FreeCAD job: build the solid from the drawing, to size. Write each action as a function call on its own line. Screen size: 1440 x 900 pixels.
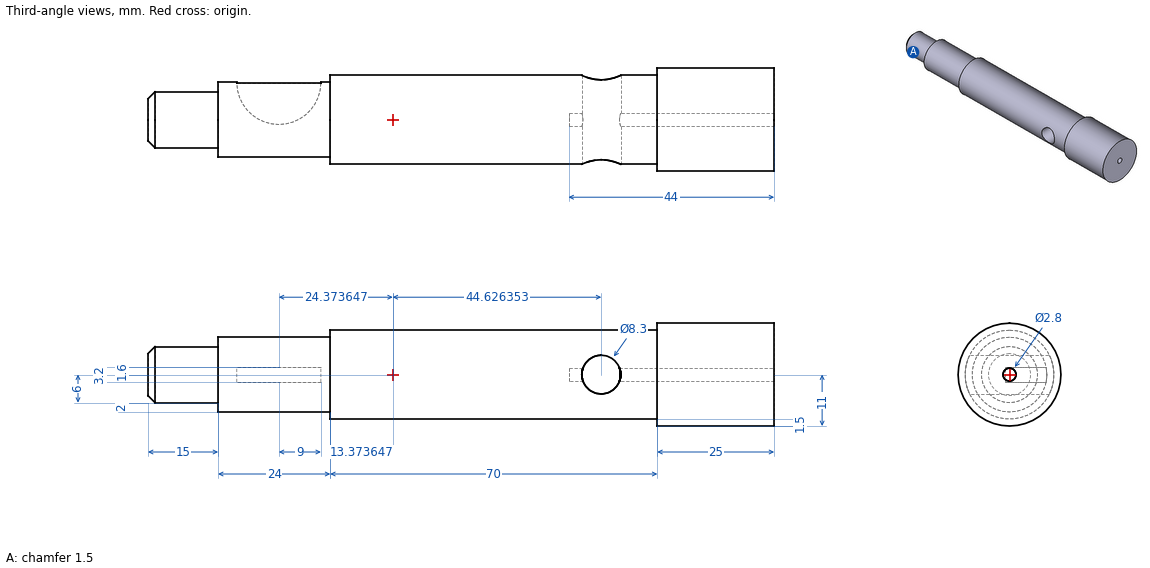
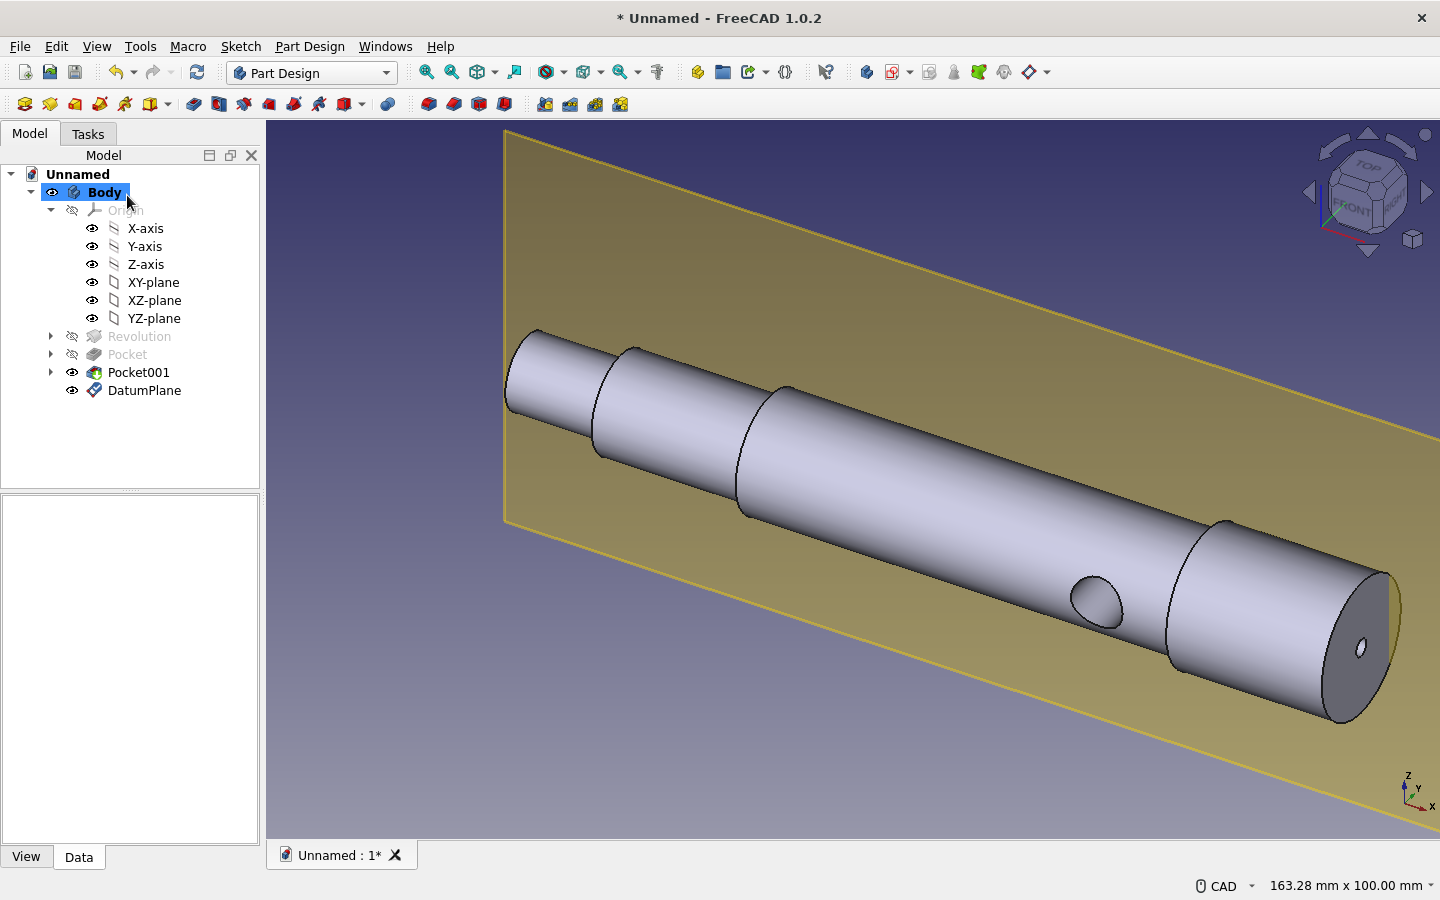
click(117, 390)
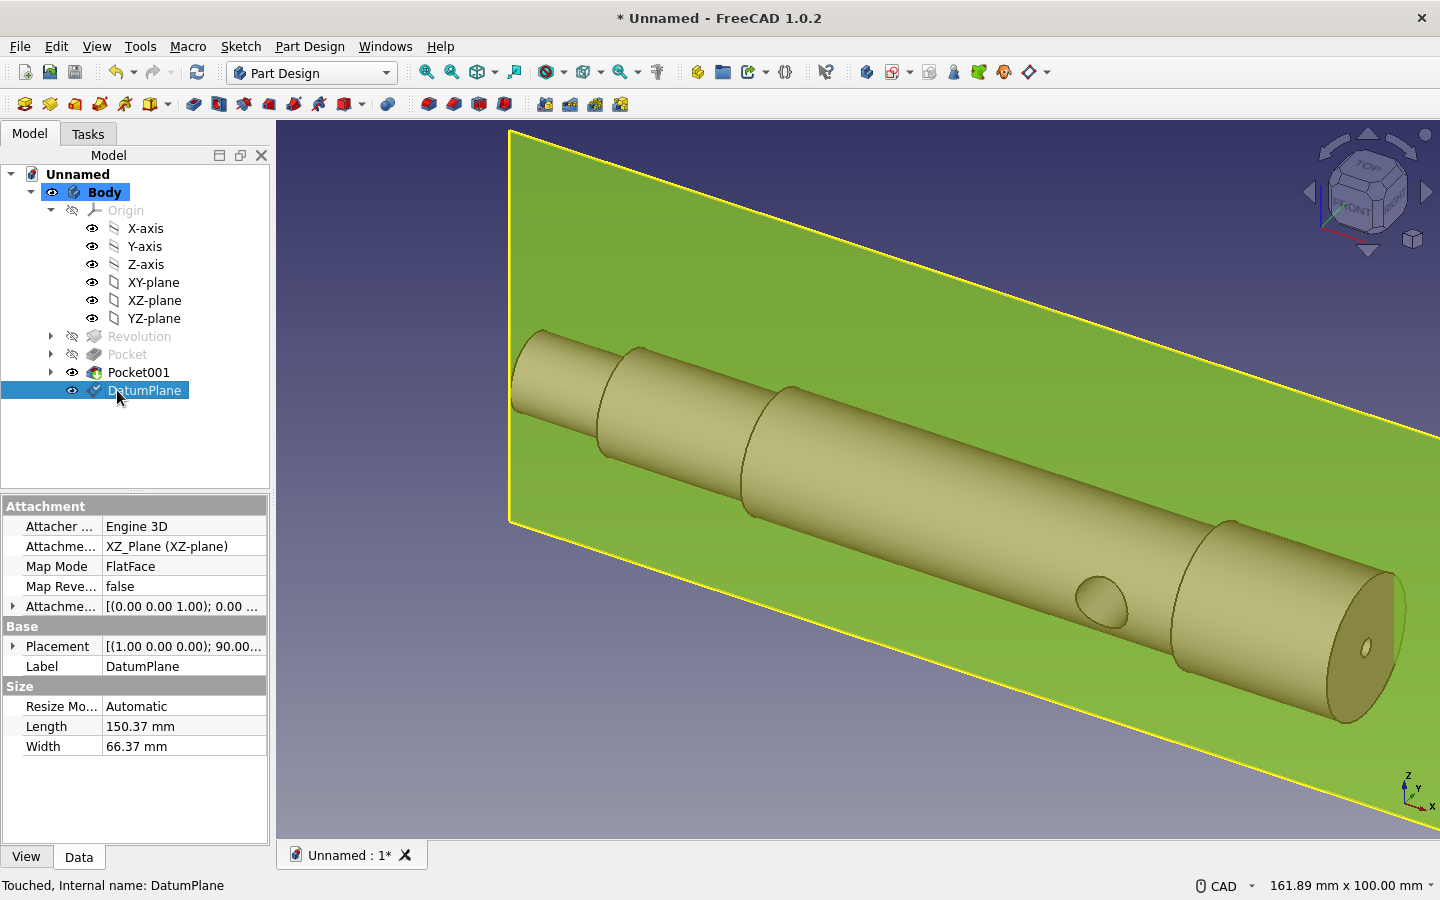
click(892, 72)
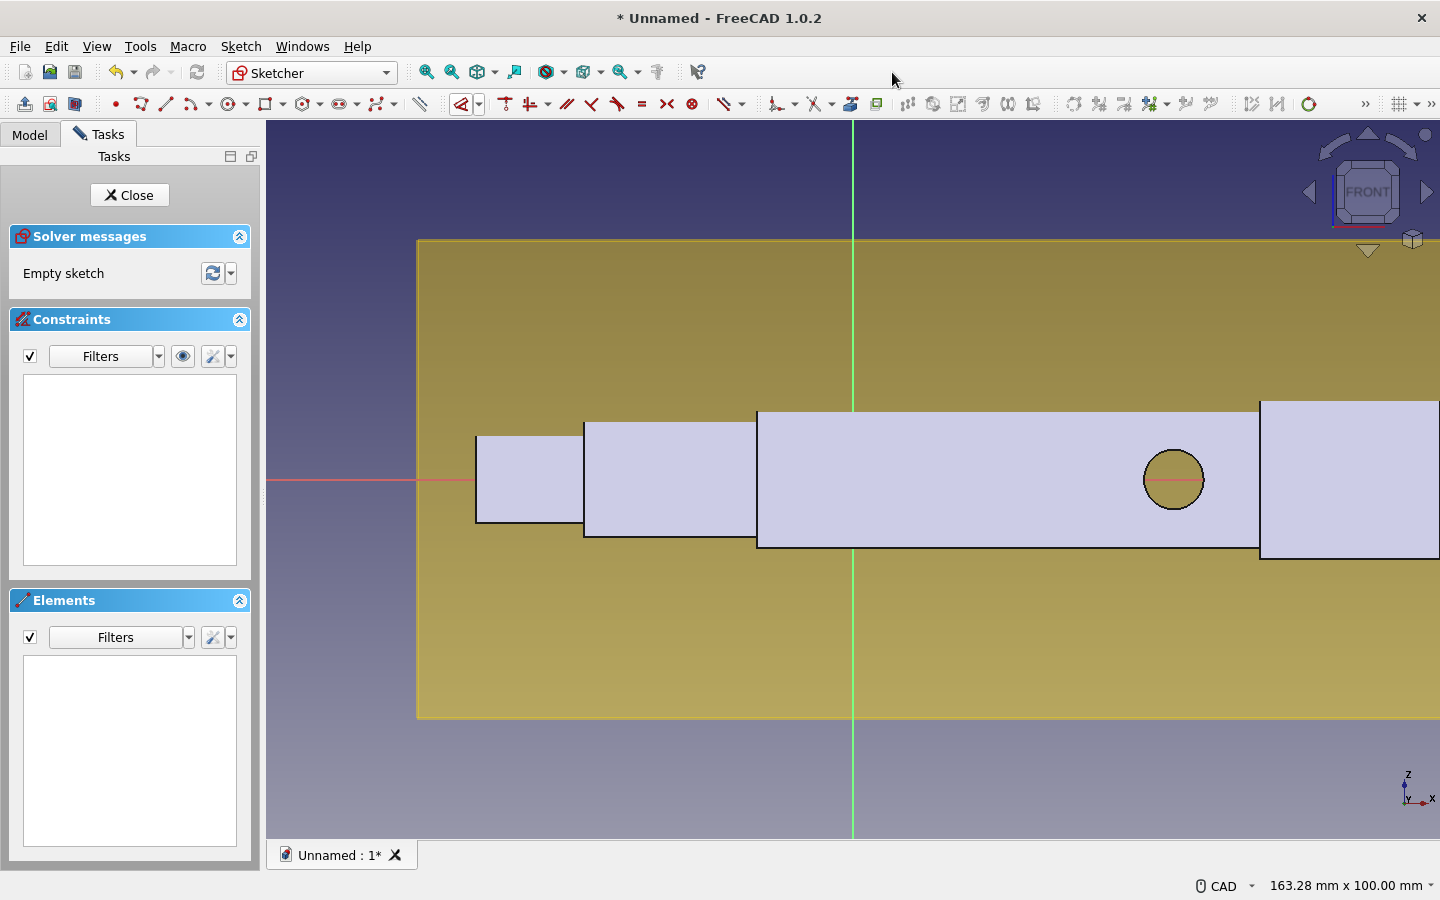
click(75, 104)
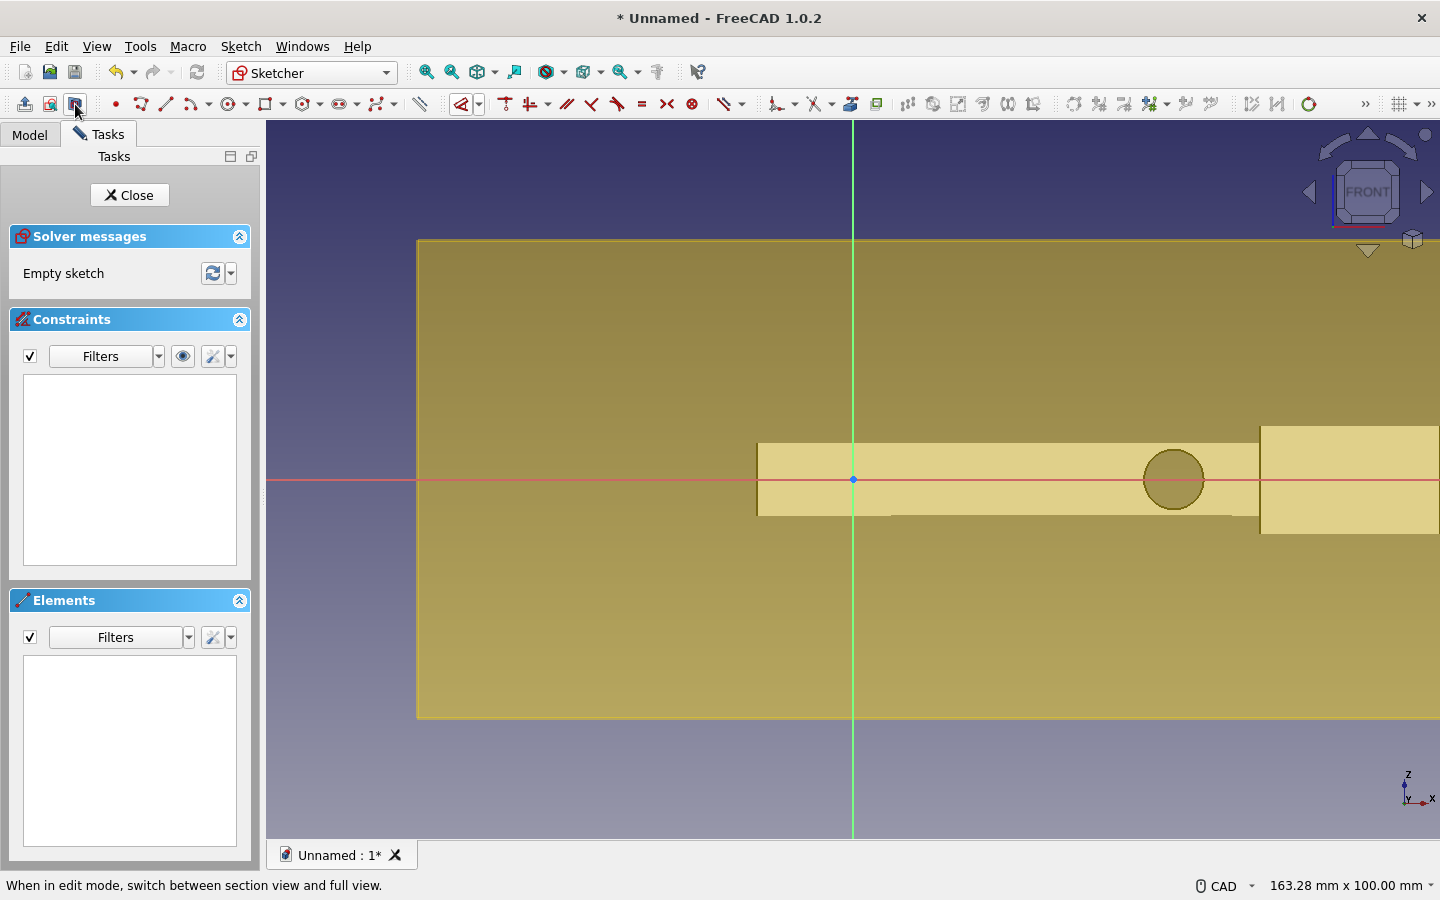
scroll(703, 485, up, 12)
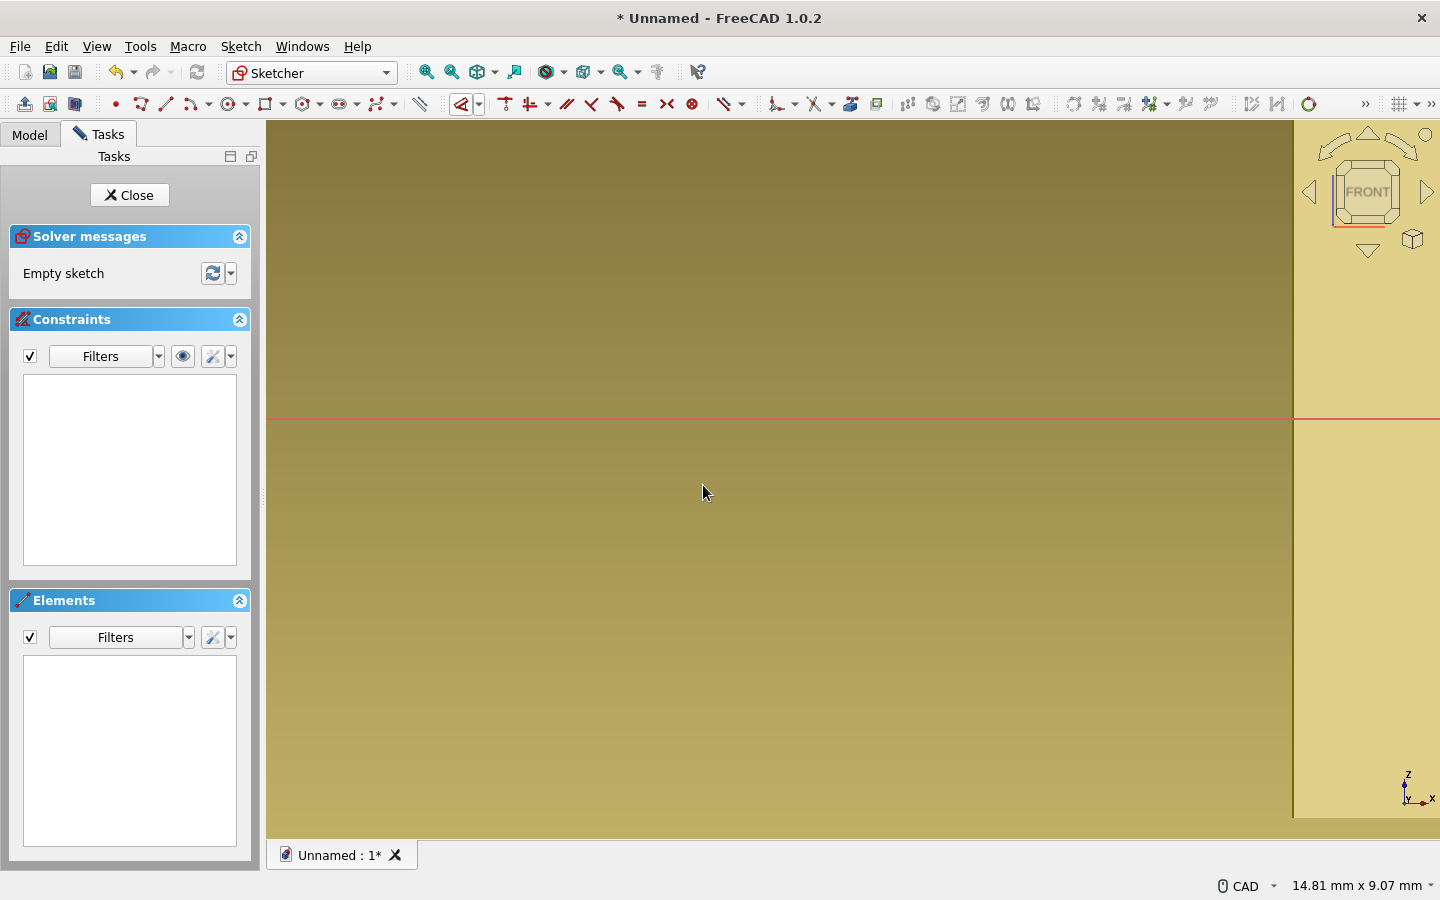
click(264, 104)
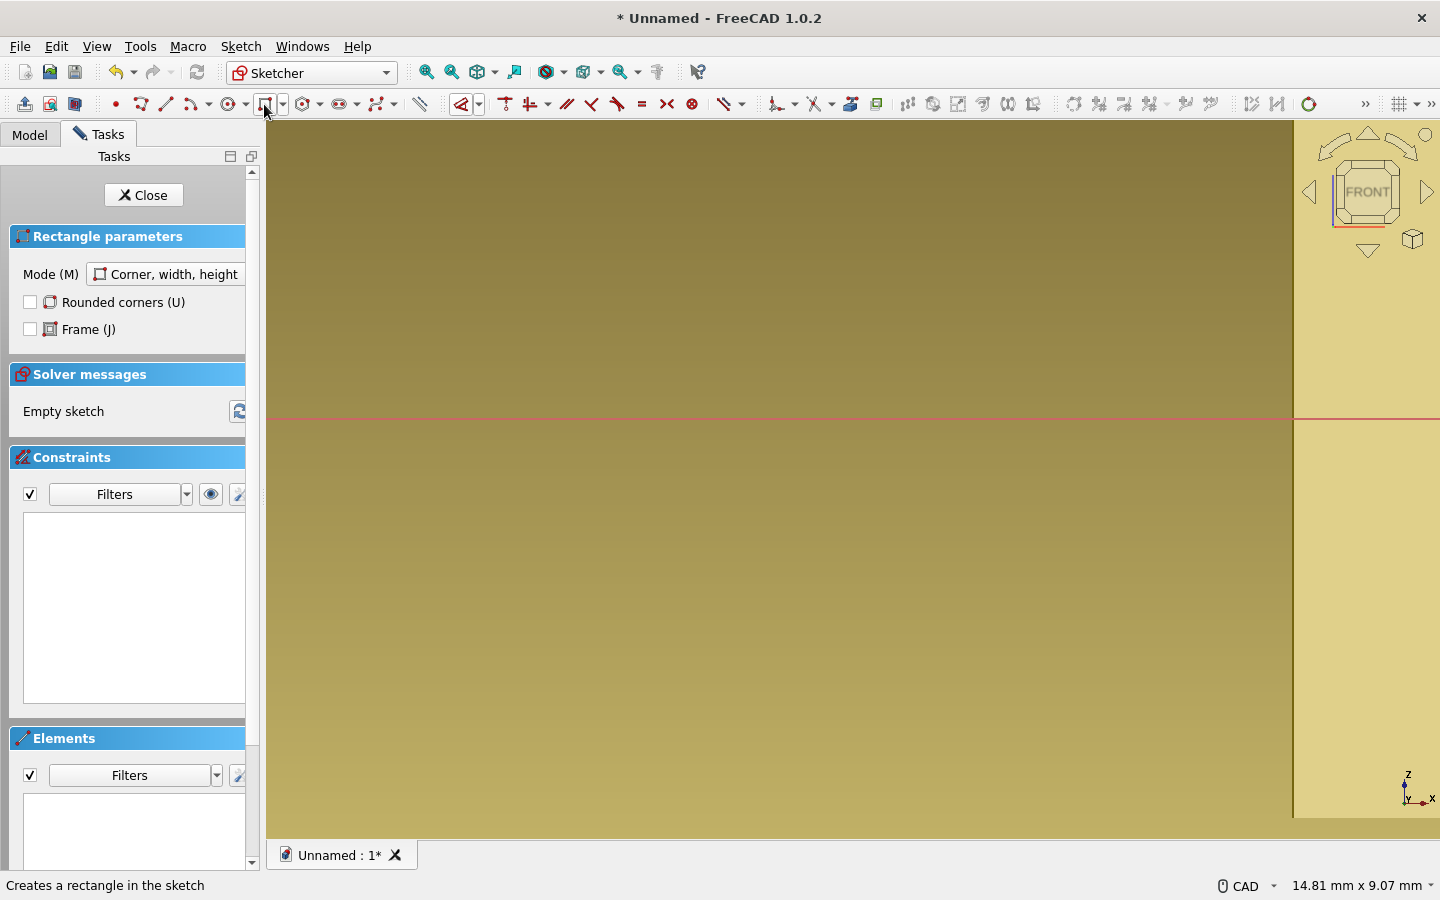
click(421, 292)
click(1134, 546)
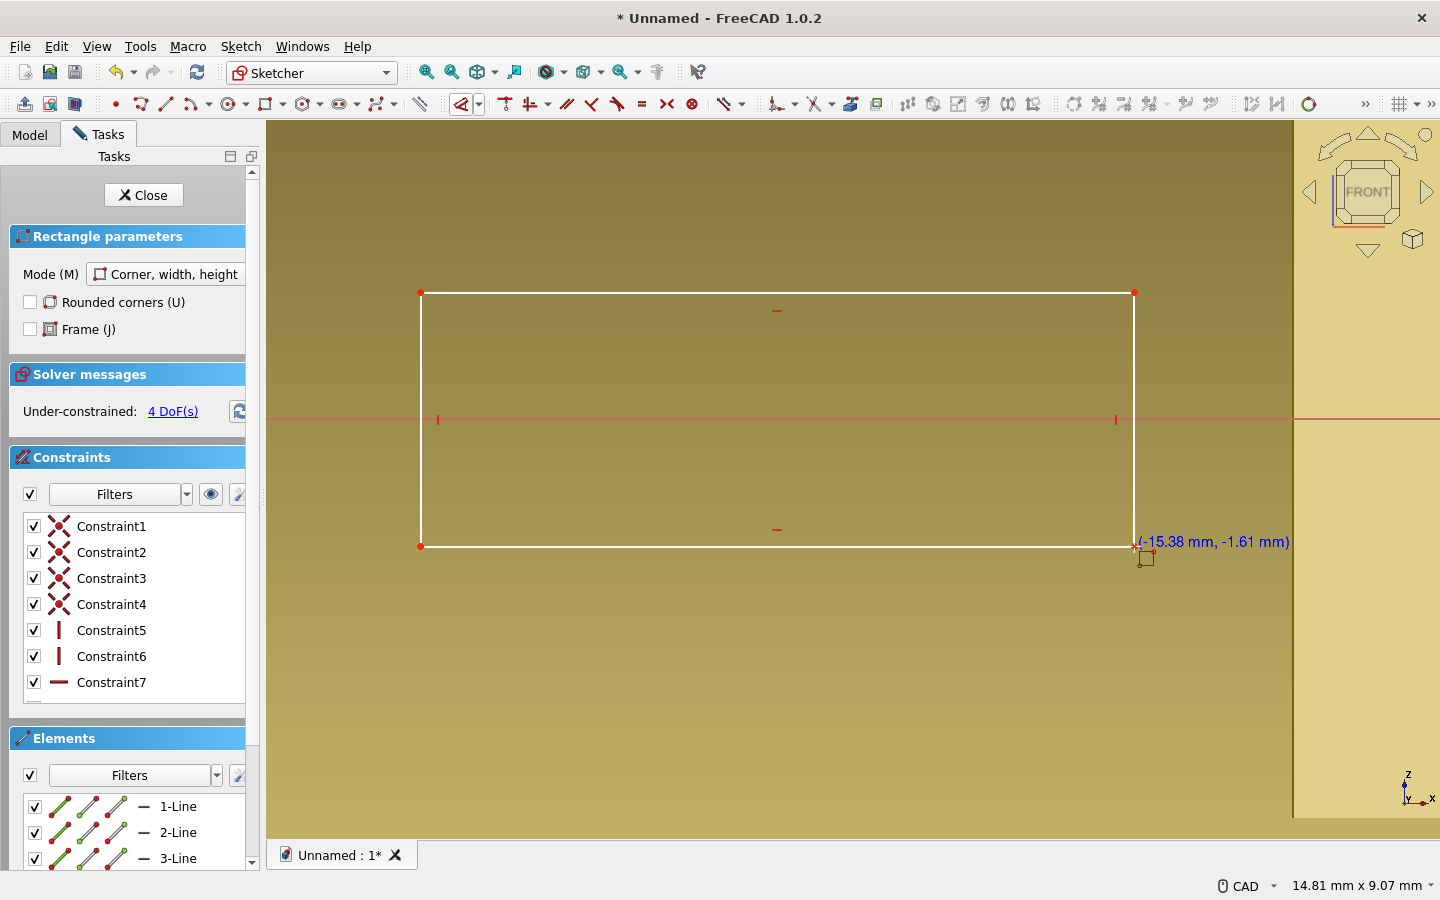
click(166, 104)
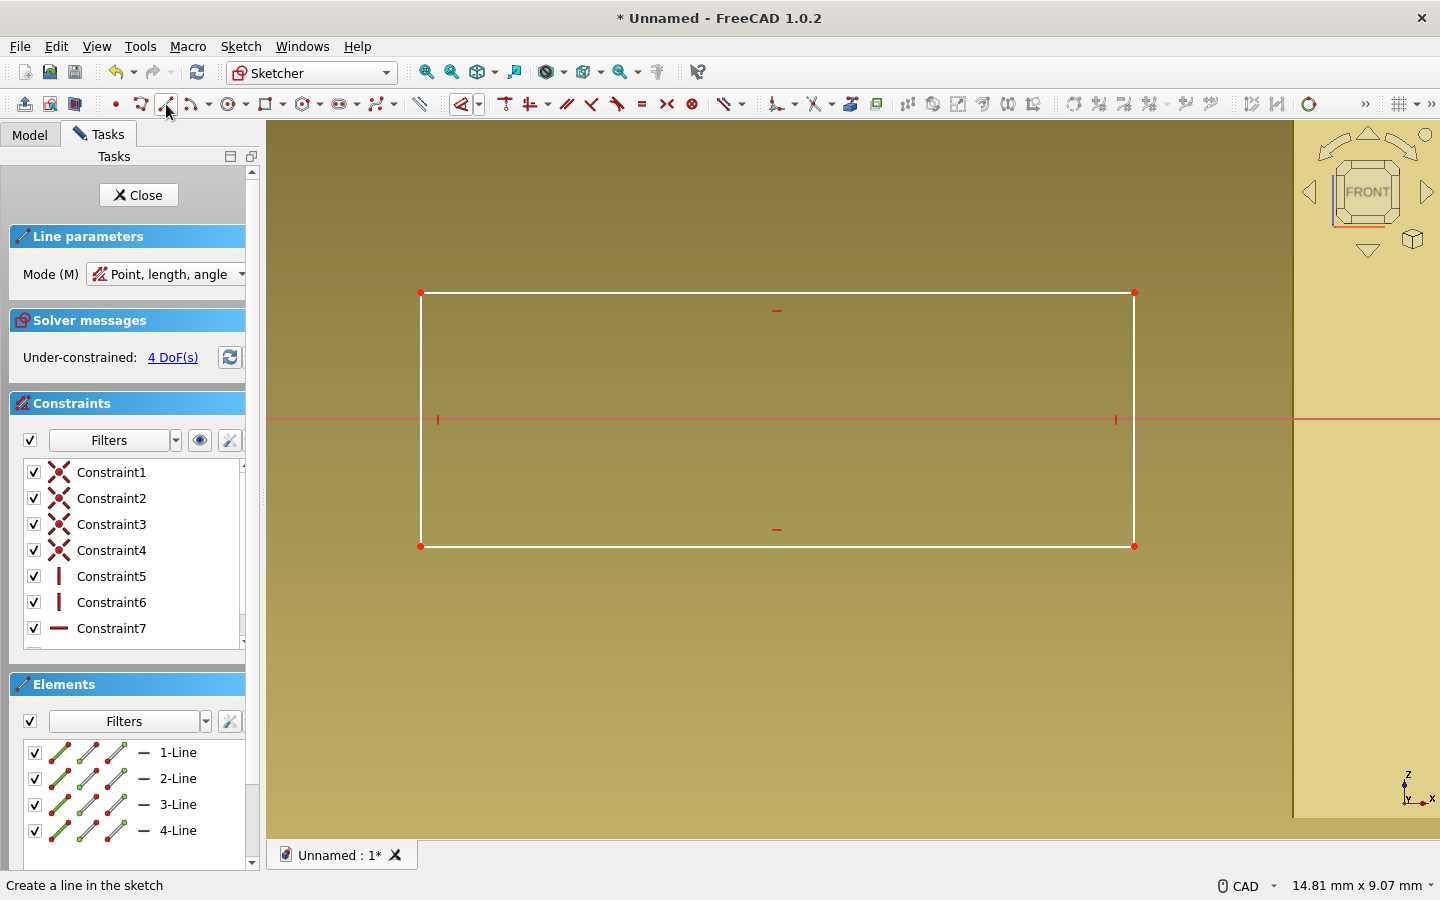
click(421, 575)
click(421, 660)
key(Escape)